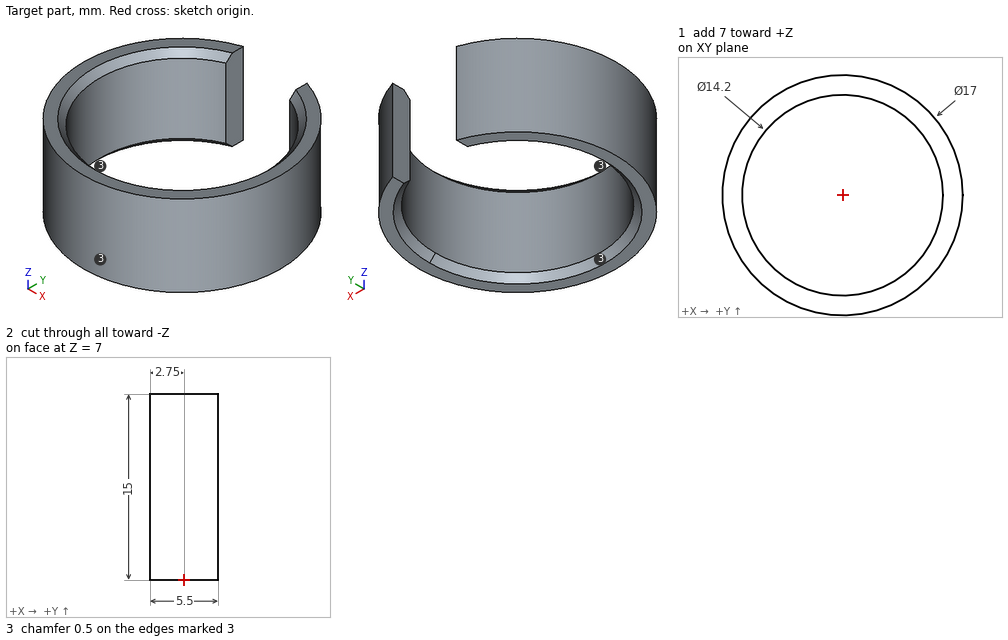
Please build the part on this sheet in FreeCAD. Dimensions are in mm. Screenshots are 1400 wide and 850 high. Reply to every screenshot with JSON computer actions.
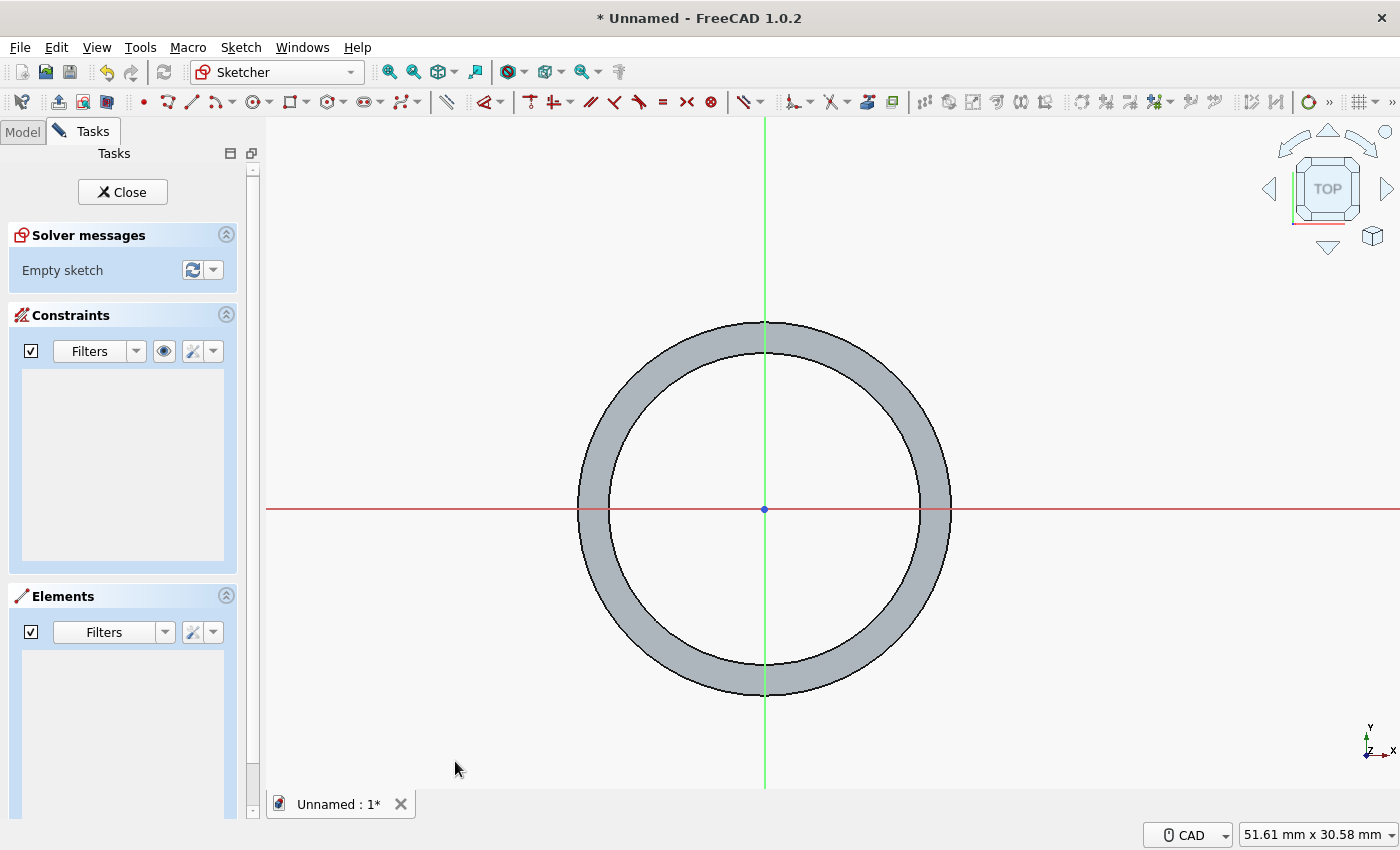
{"action": "left_click", "coordinate": [290, 102]}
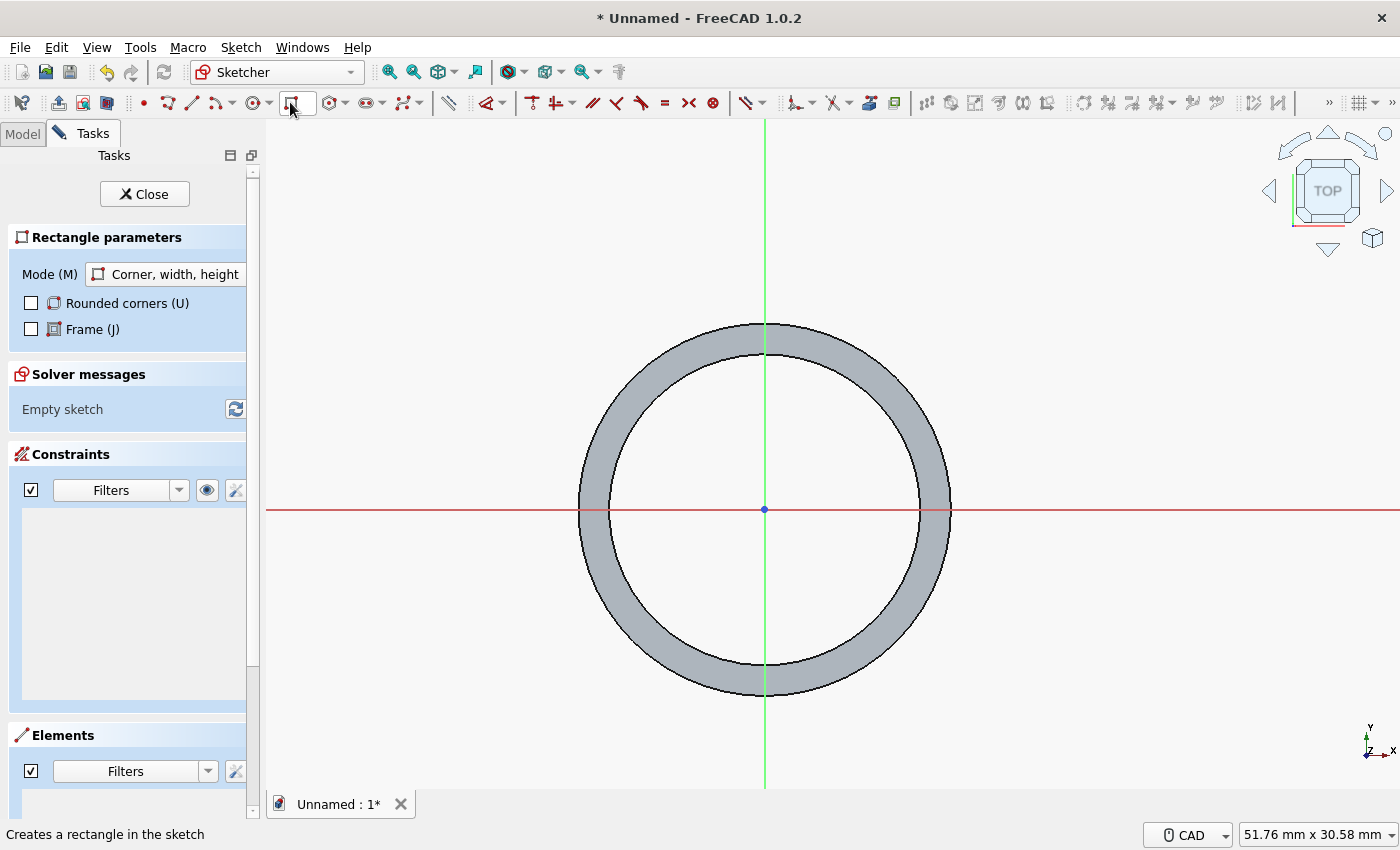
{"action": "left_click", "coordinate": [704, 181]}
{"action": "left_click", "coordinate": [825, 510]}
{"action": "key", "text": "Escape"}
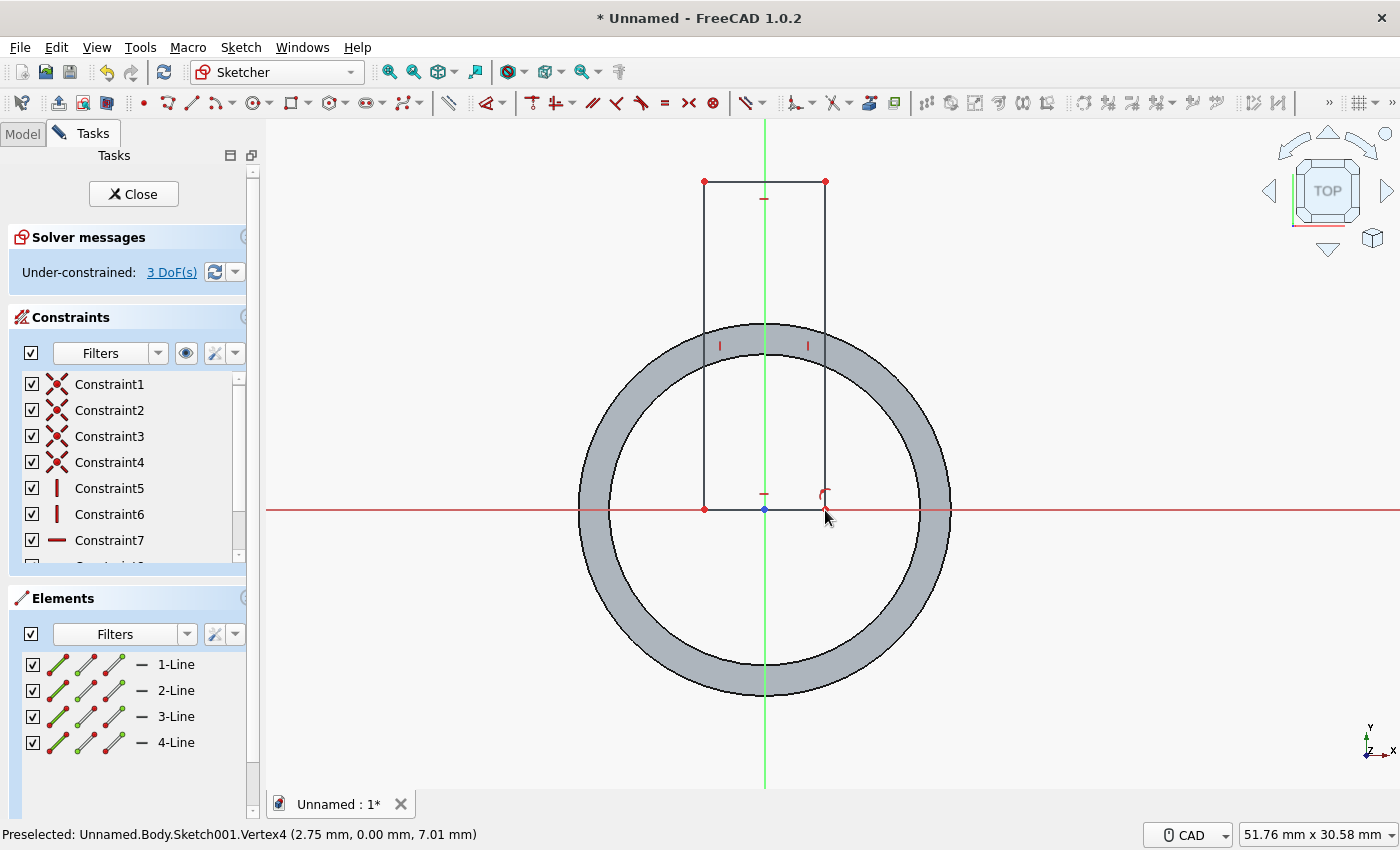
{"action": "left_click", "coordinate": [486, 104]}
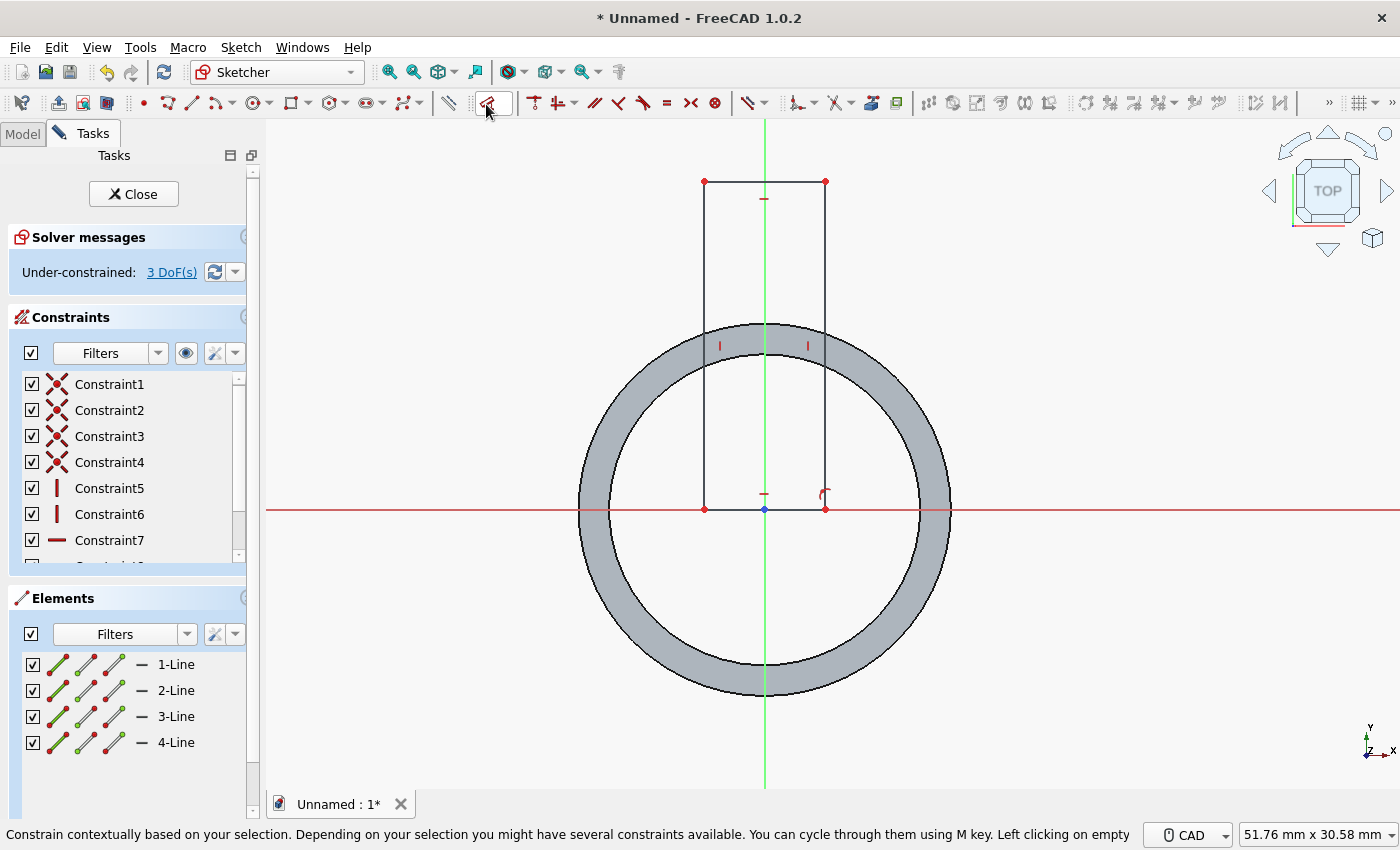
{"action": "left_click", "coordinate": [704, 280]}
{"action": "left_click", "coordinate": [670, 346]}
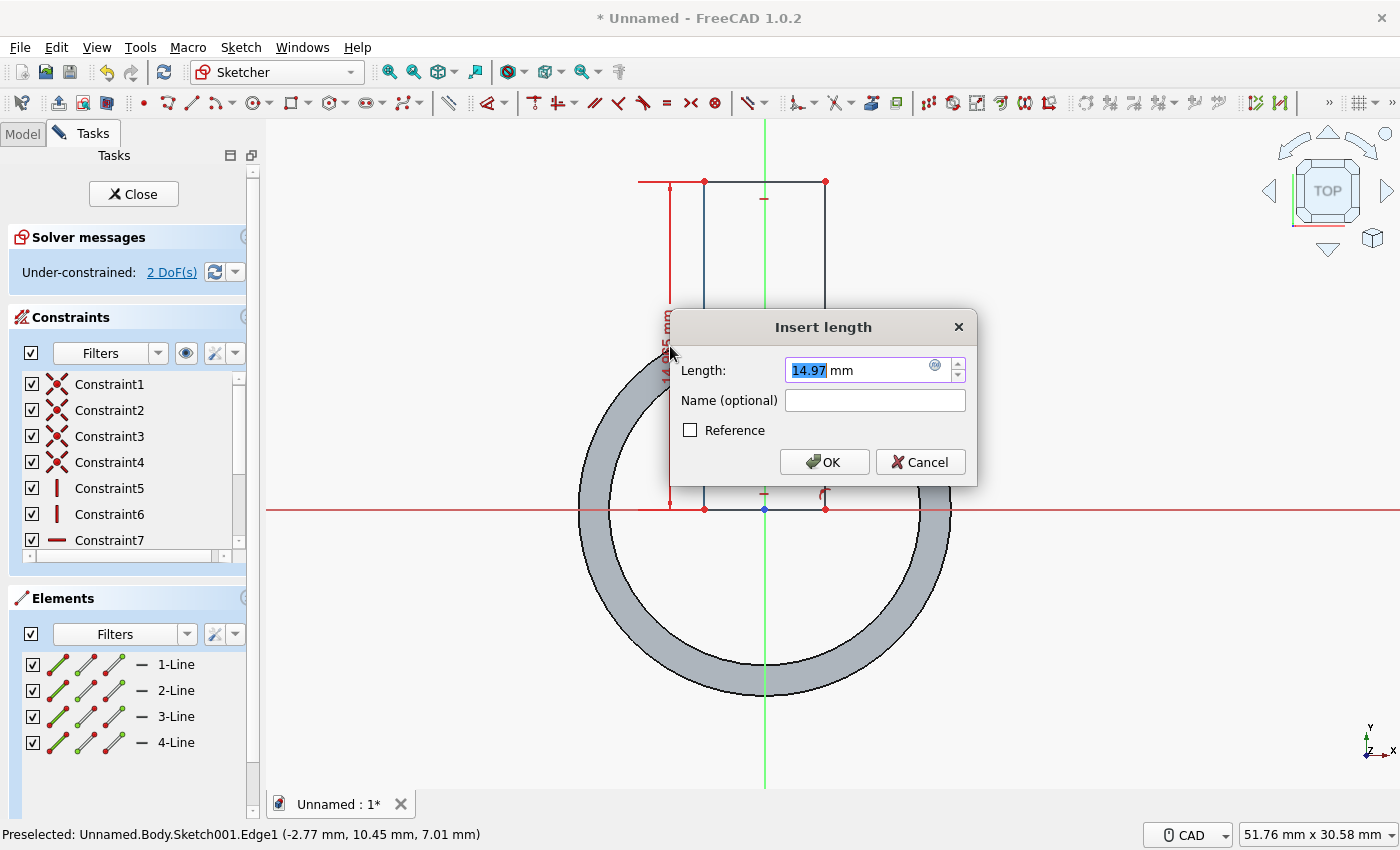
{"action": "type", "text": "15"}
{"action": "key", "text": "Return"}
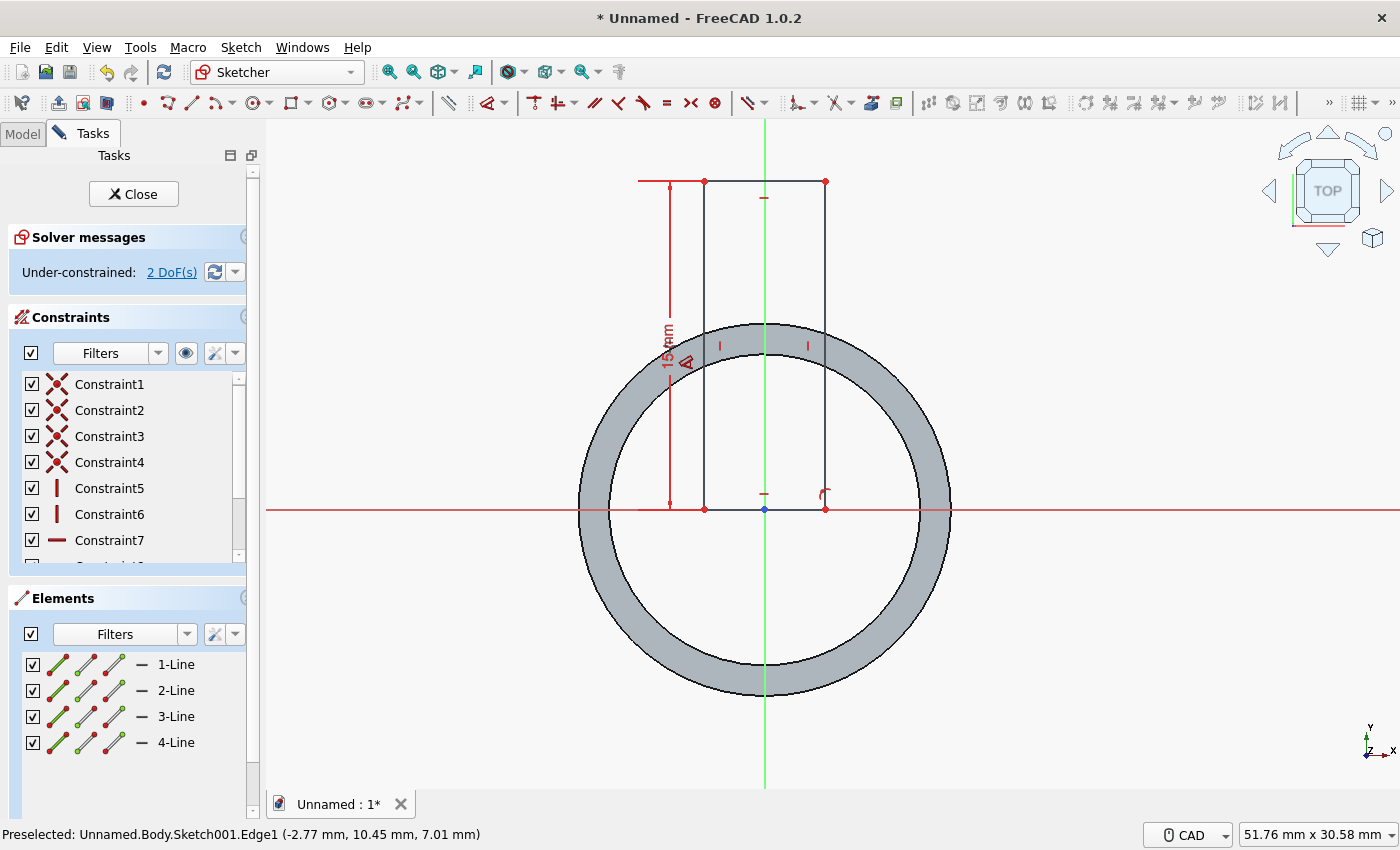
{"action": "left_click", "coordinate": [740, 510]}
{"action": "left_click", "coordinate": [737, 544]}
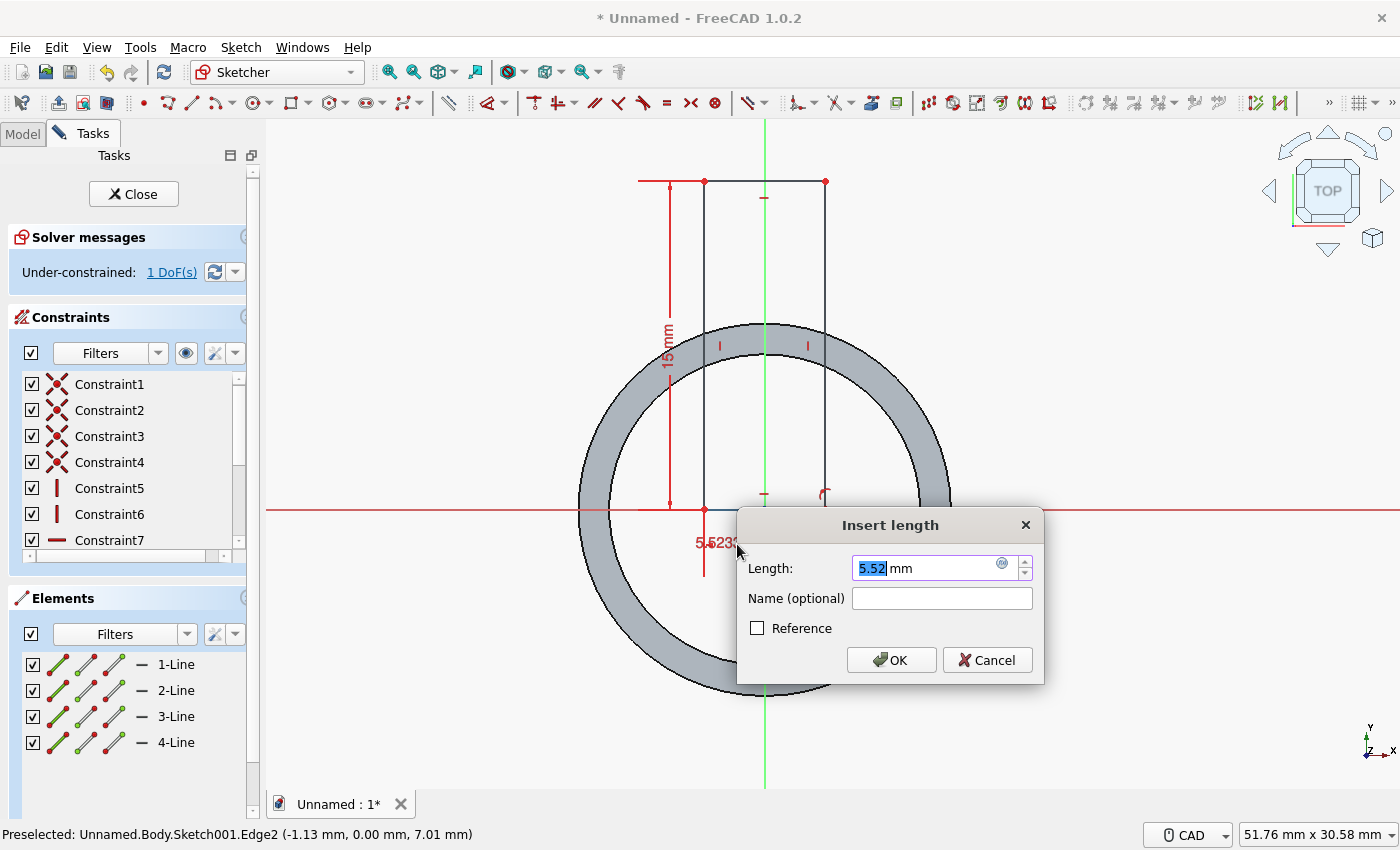
{"action": "type", "text": "5.5"}
{"action": "key", "text": "Return"}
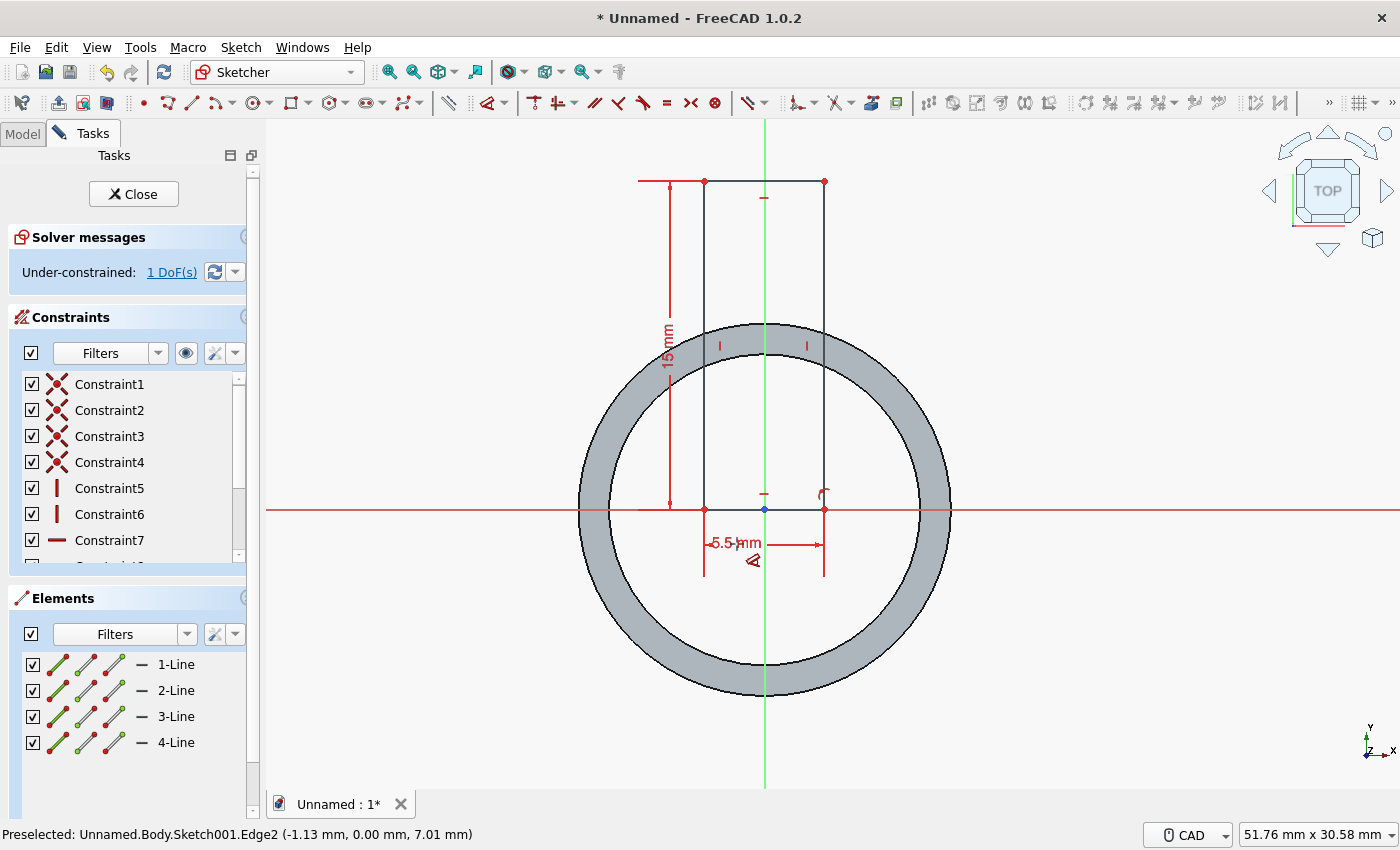
{"action": "left_click", "coordinate": [704, 181]}
{"action": "left_click", "coordinate": [734, 147]}